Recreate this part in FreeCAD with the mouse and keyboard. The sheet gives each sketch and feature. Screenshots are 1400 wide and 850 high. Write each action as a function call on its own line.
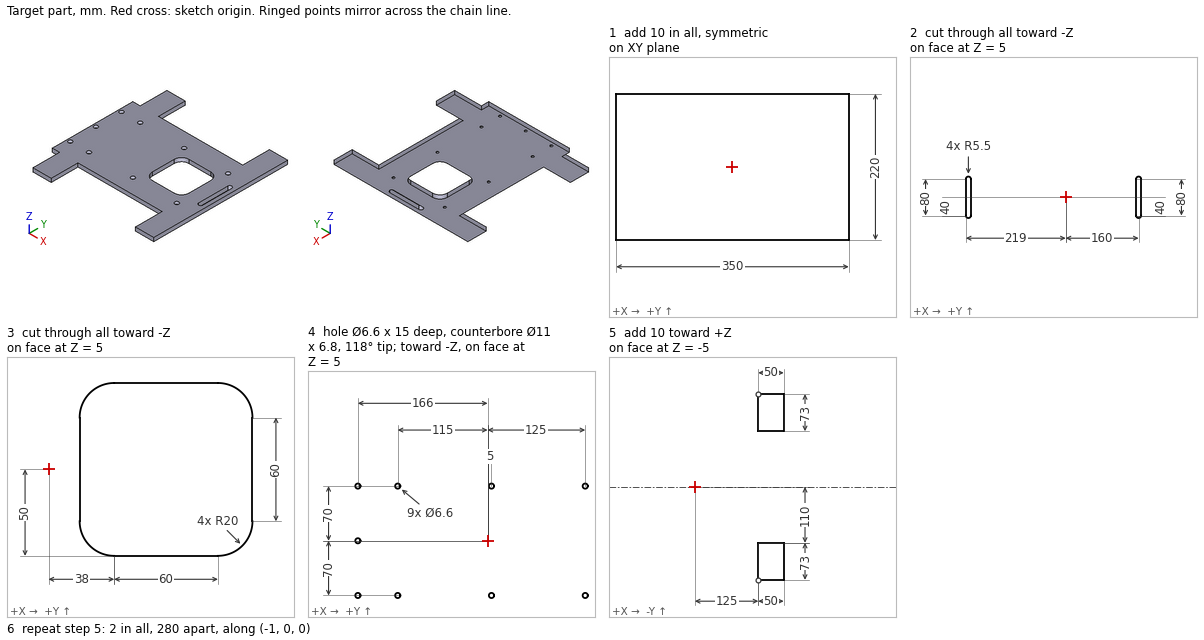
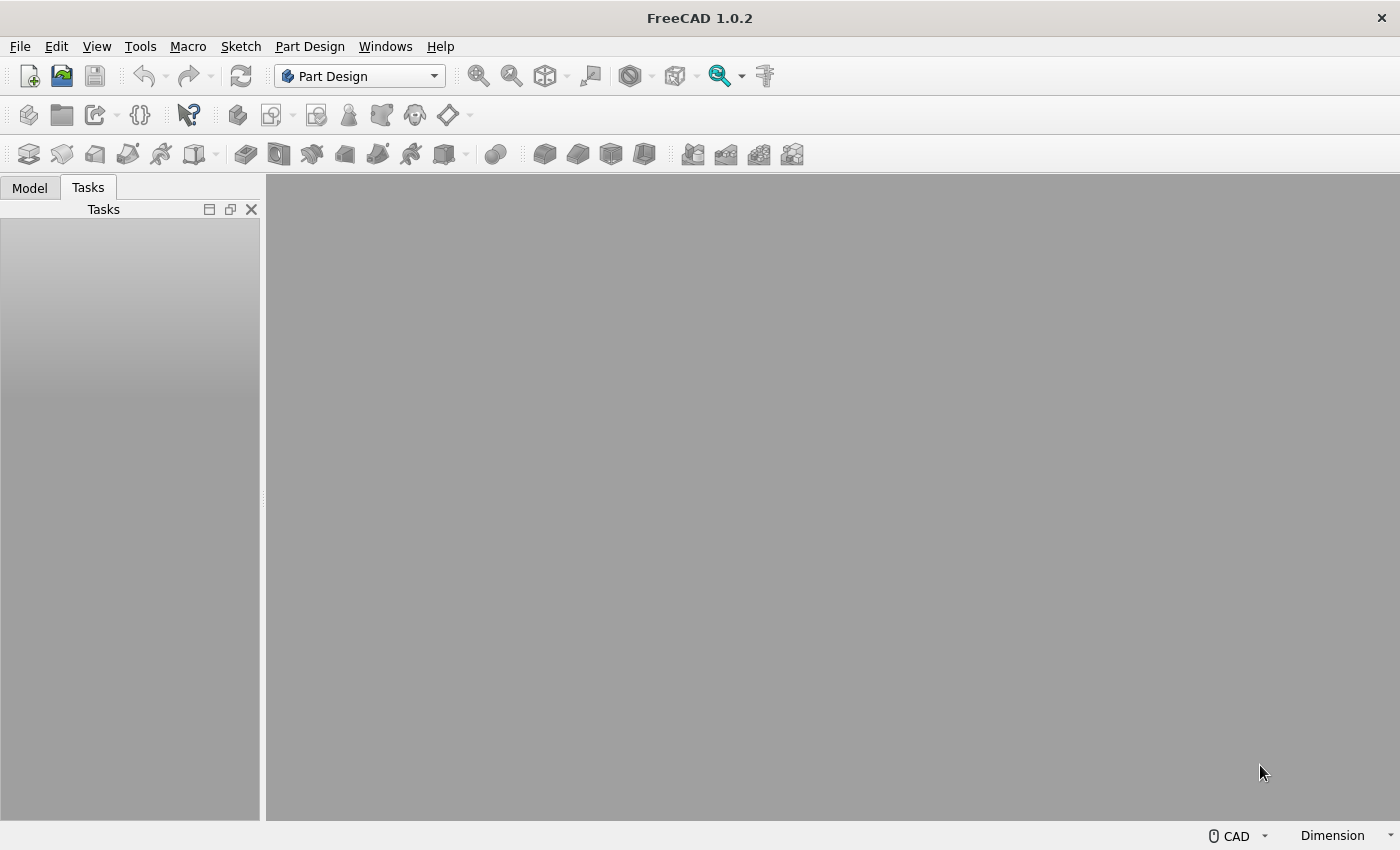
click(29, 76)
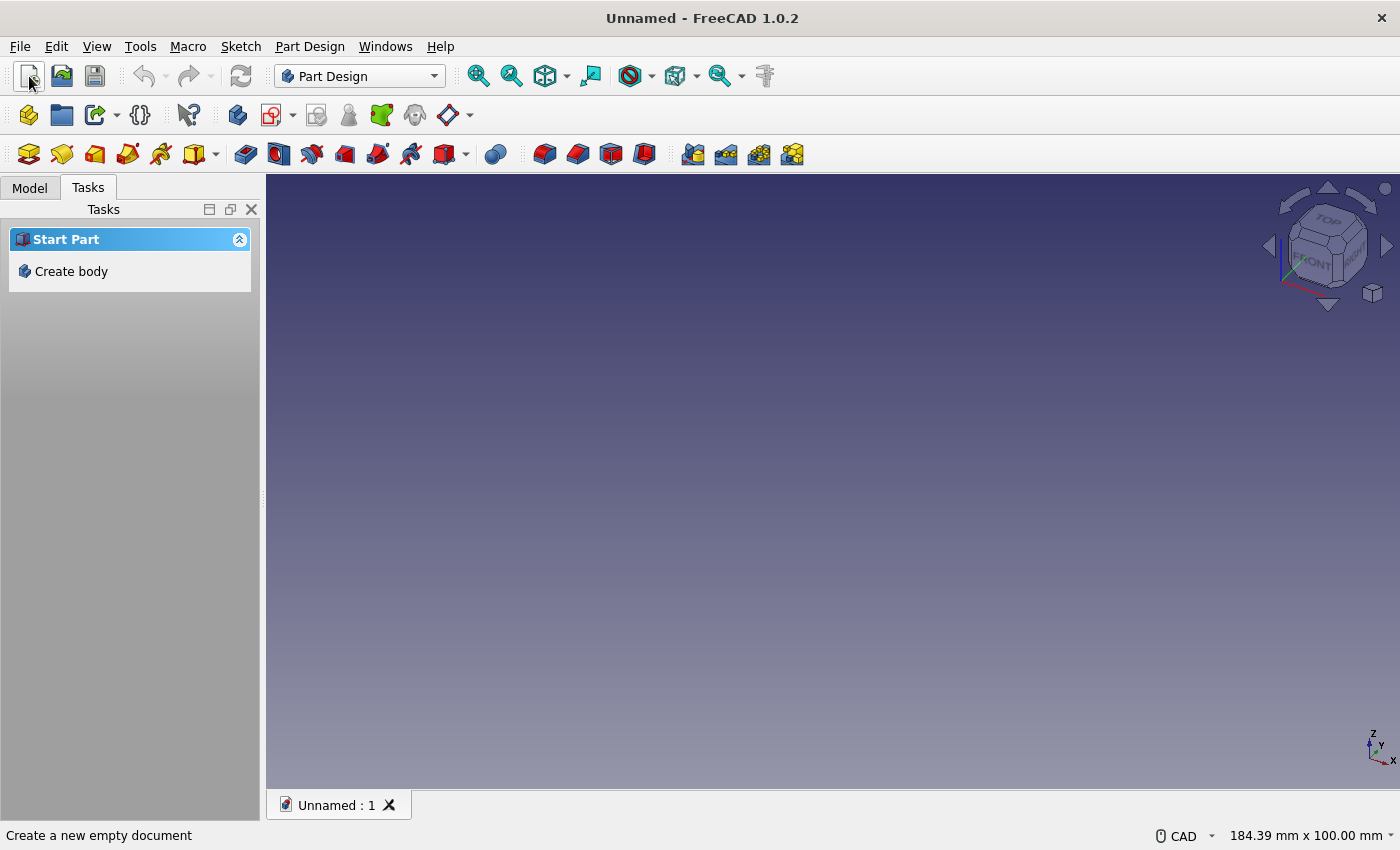
click(270, 116)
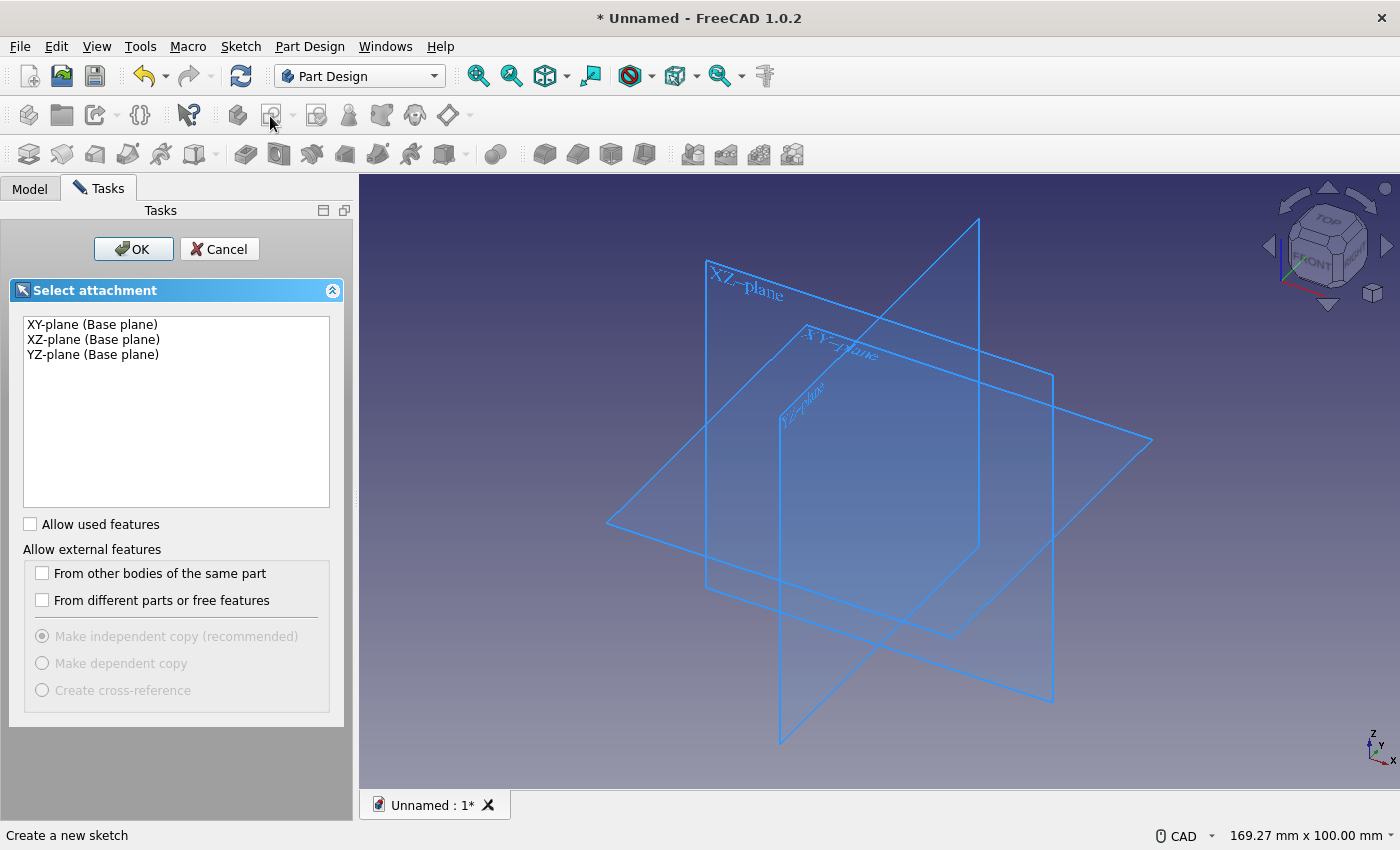
click(84, 324)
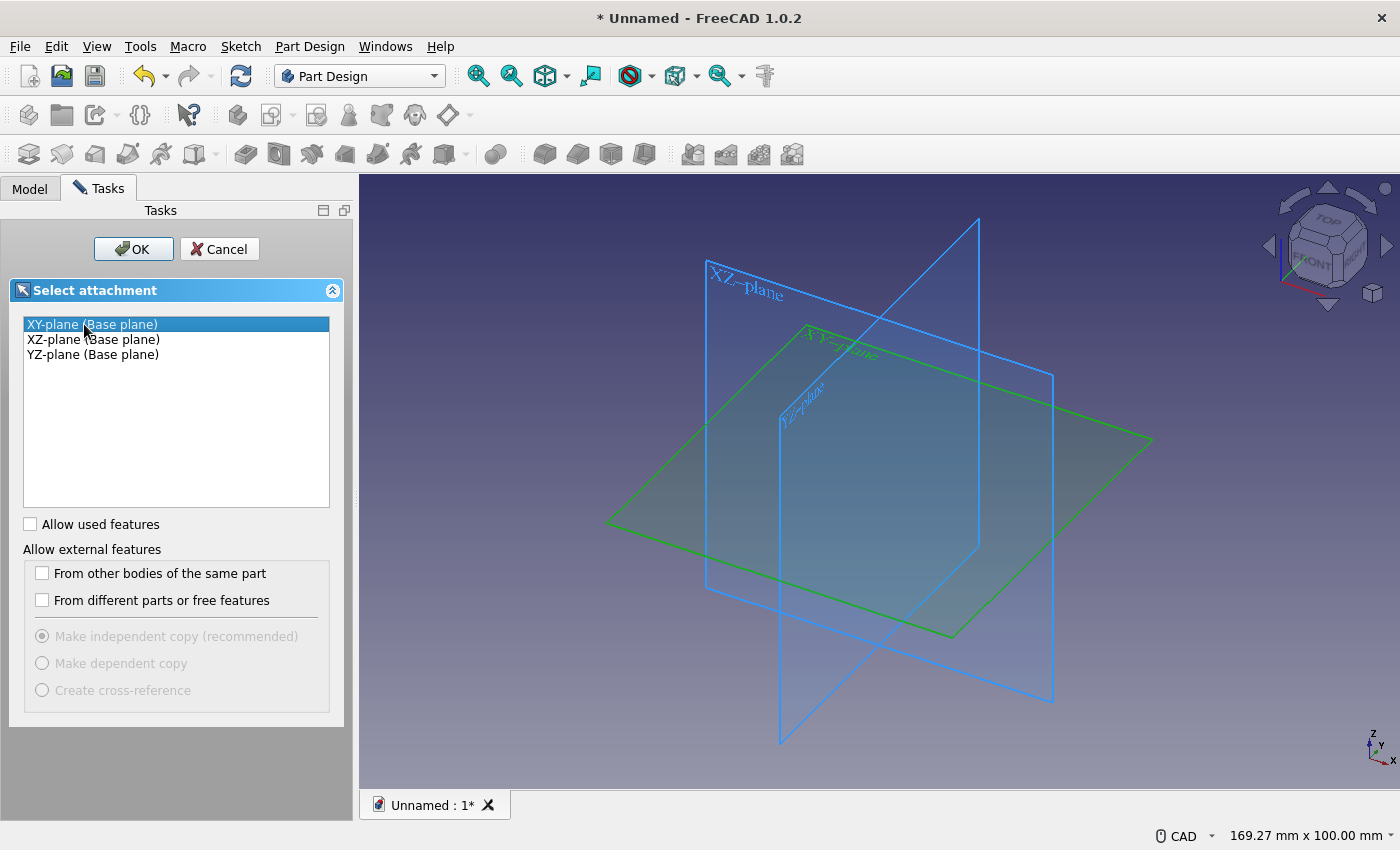
click(134, 249)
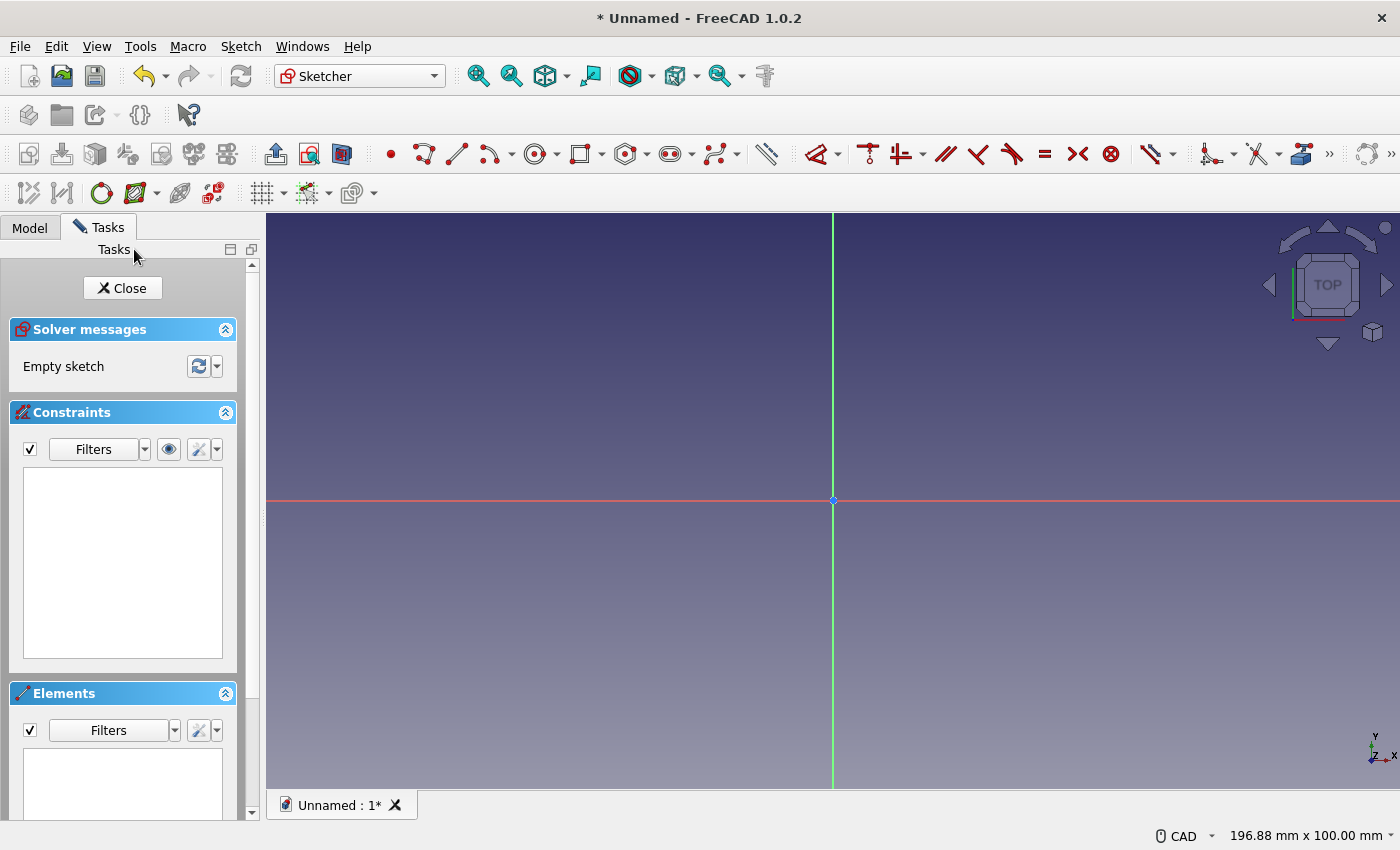
scroll(735, 501, down, 6)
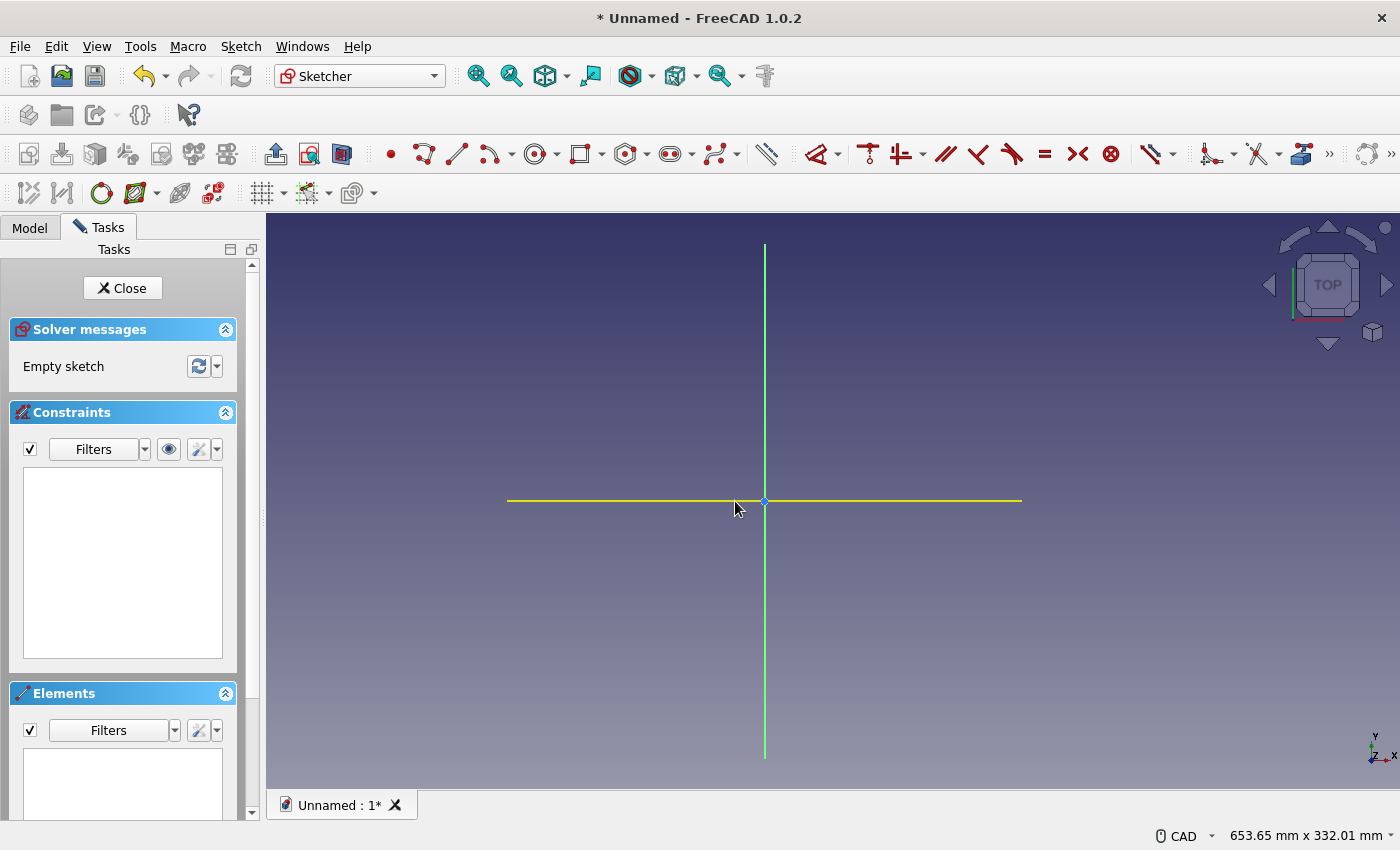
click(602, 154)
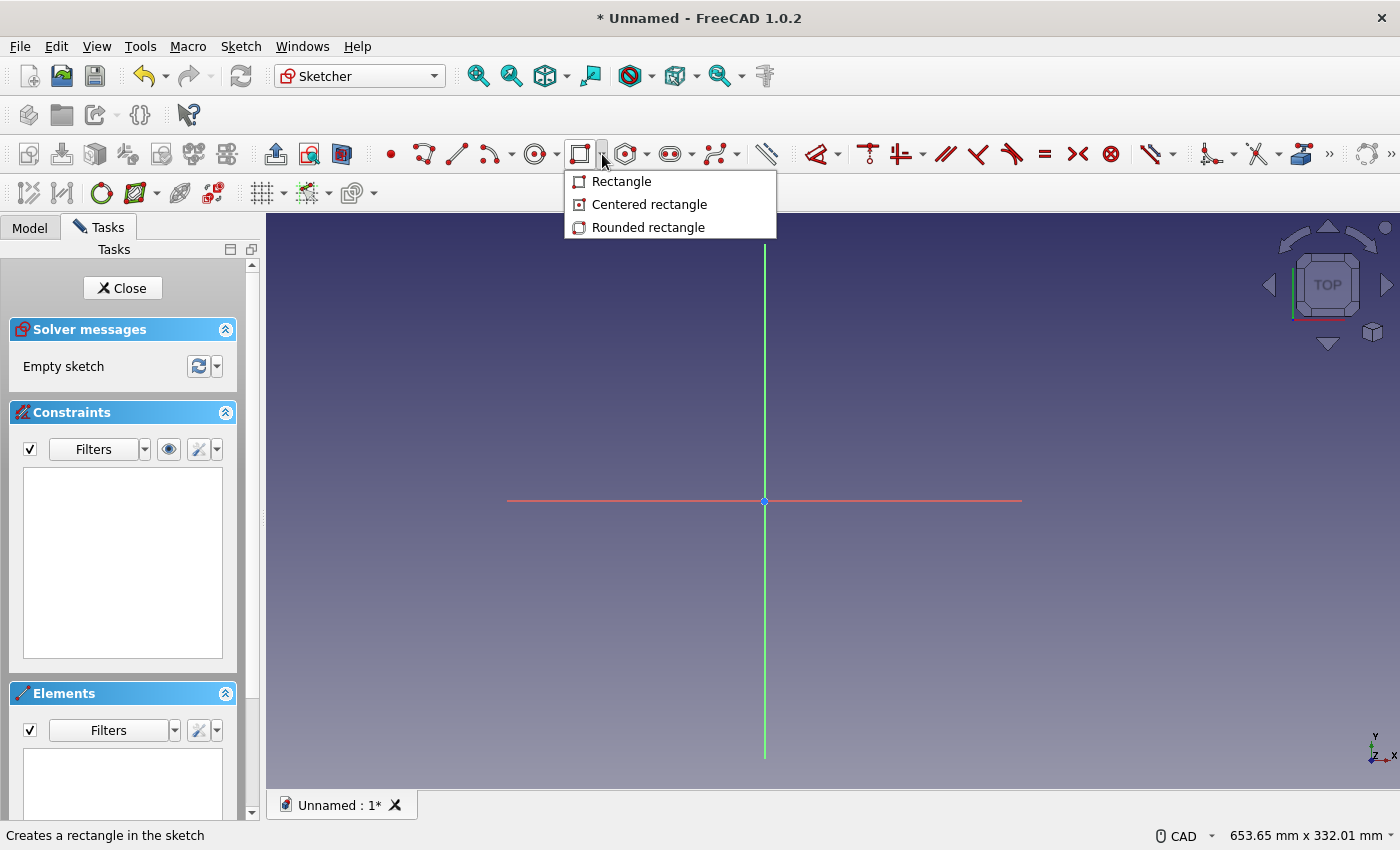
click(670, 204)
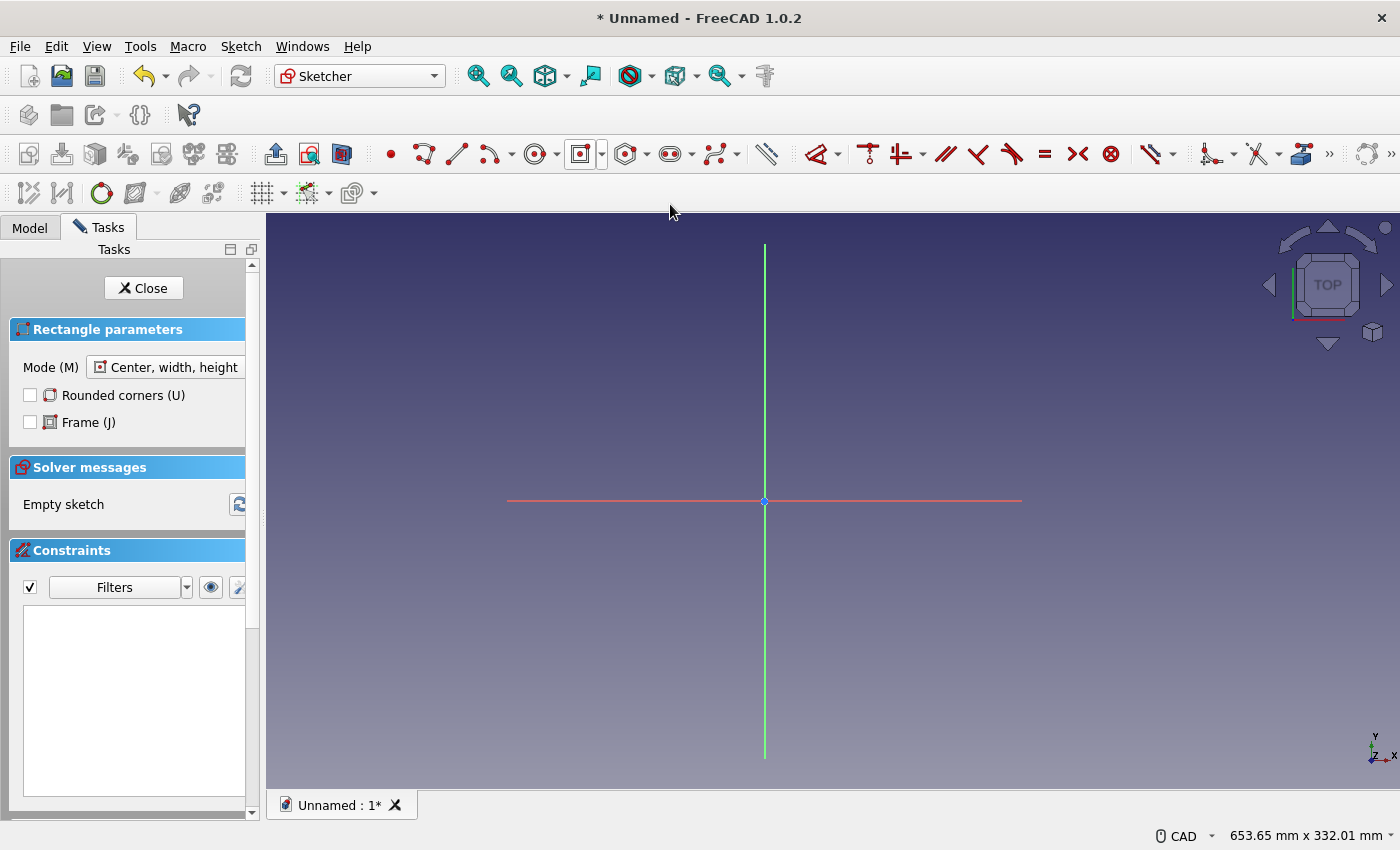
click(765, 501)
move(1068, 311)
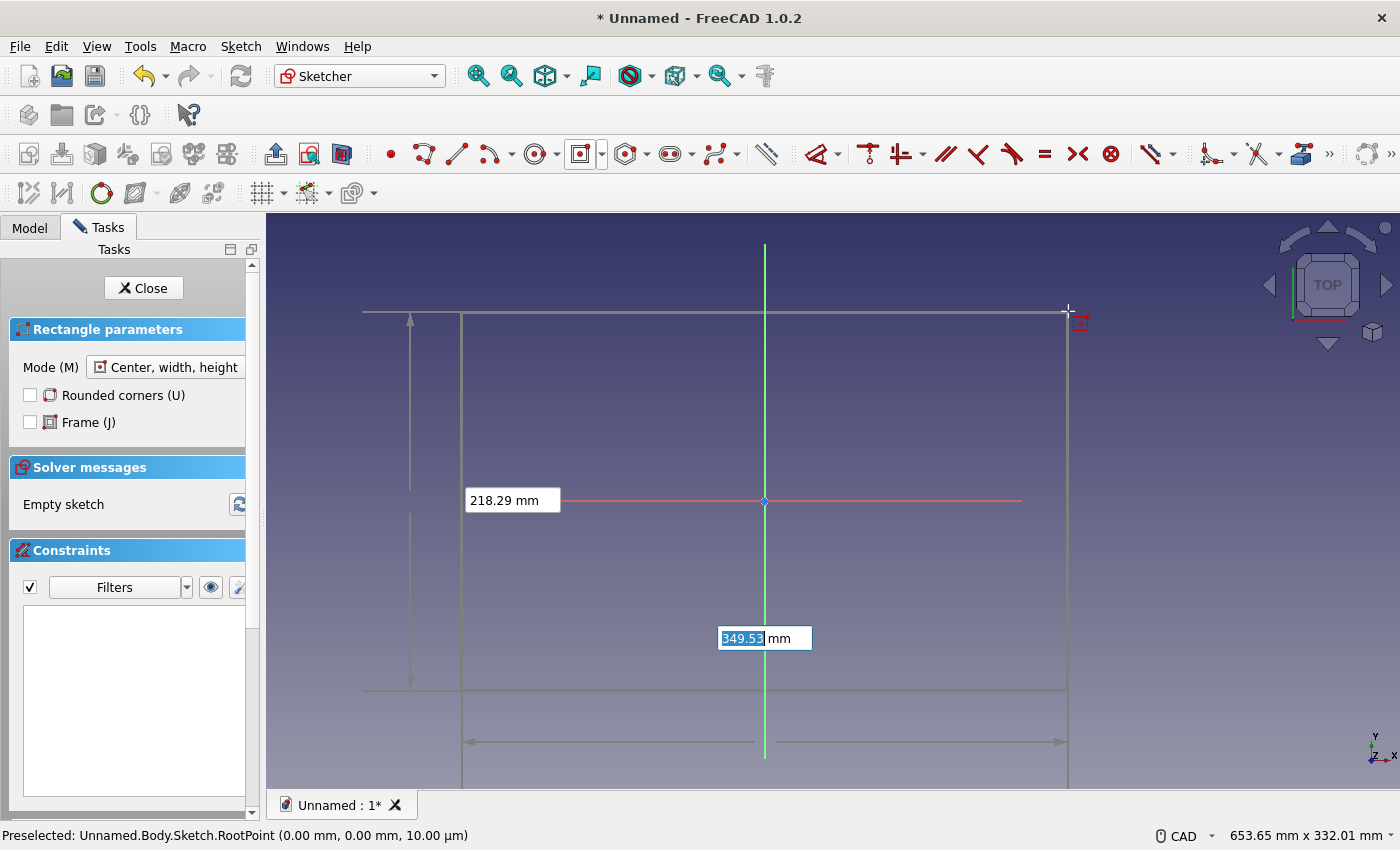
text(350)
key(Tab)
text(220)
key(Return)
key(Escape)